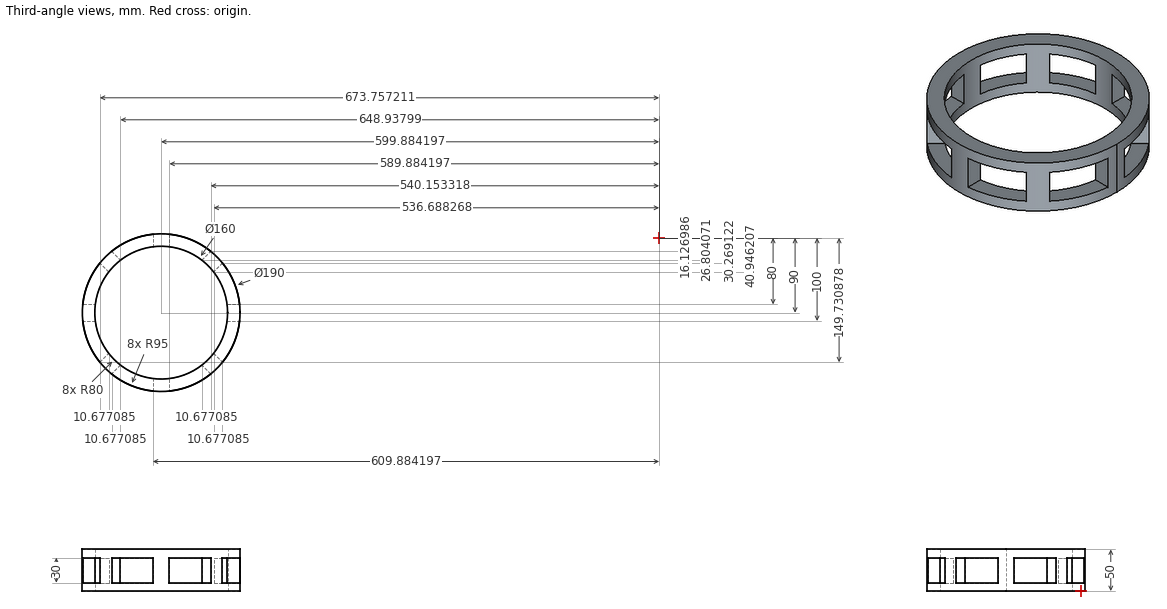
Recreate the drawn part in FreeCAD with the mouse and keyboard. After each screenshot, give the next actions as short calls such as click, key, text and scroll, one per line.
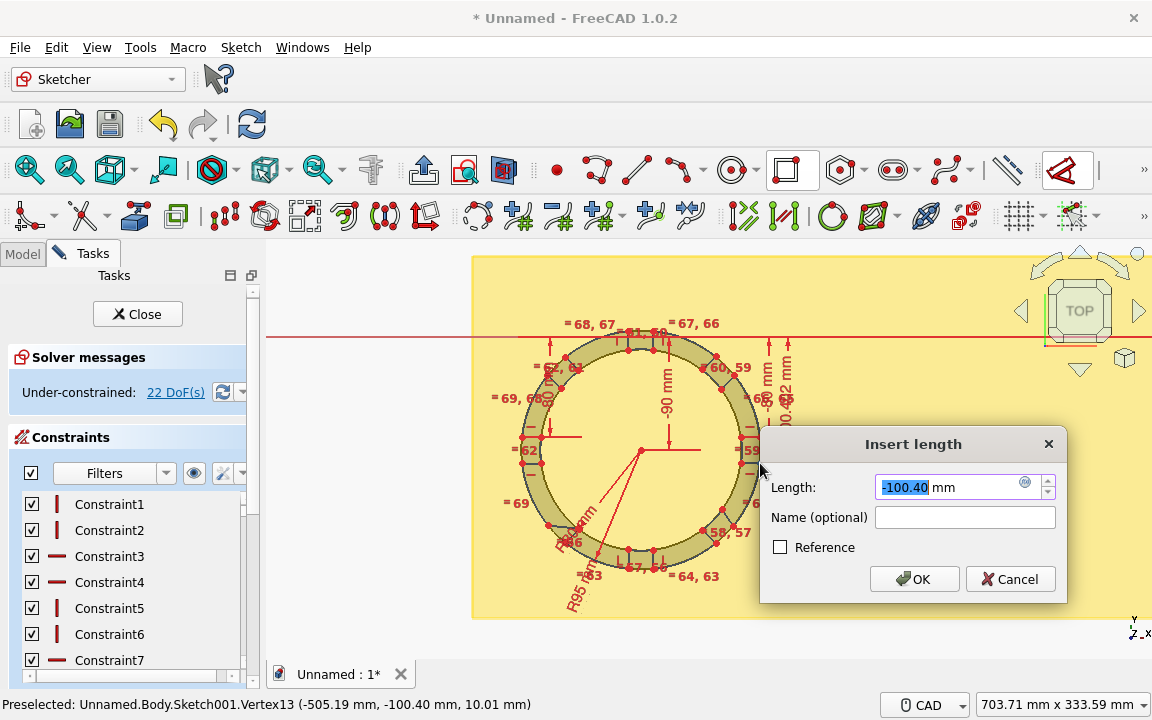
text(-100)
key(Return)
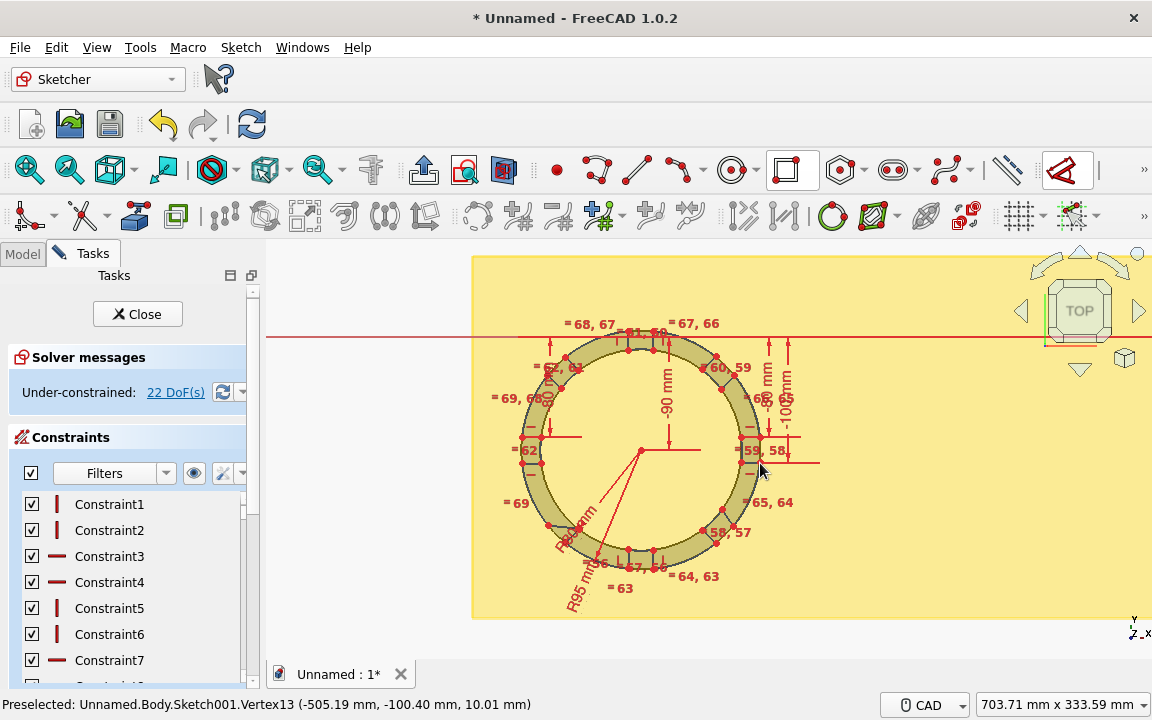
click(541, 464)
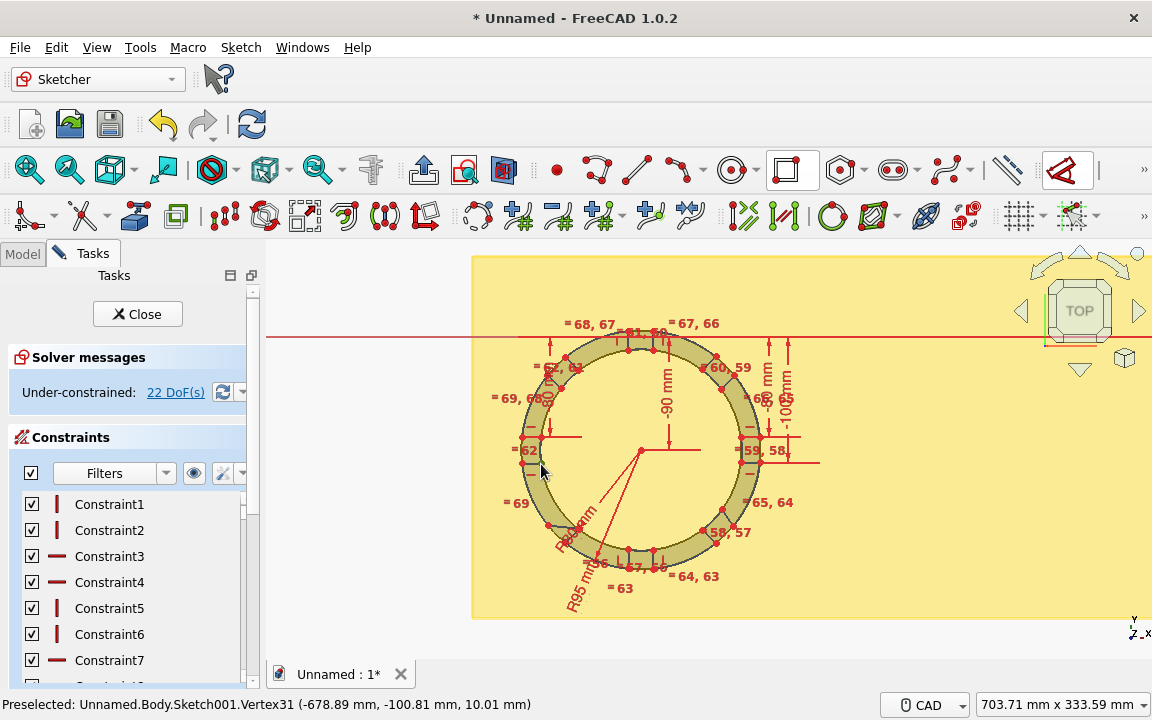
key(i)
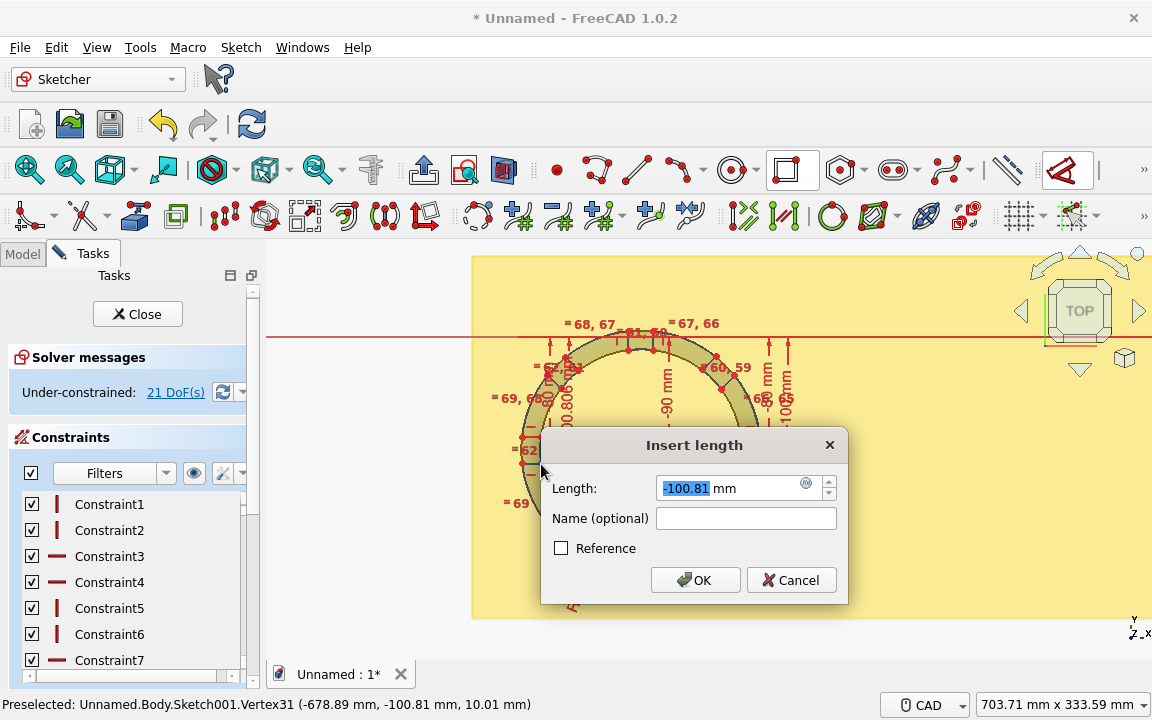
text(-100)
key(Return)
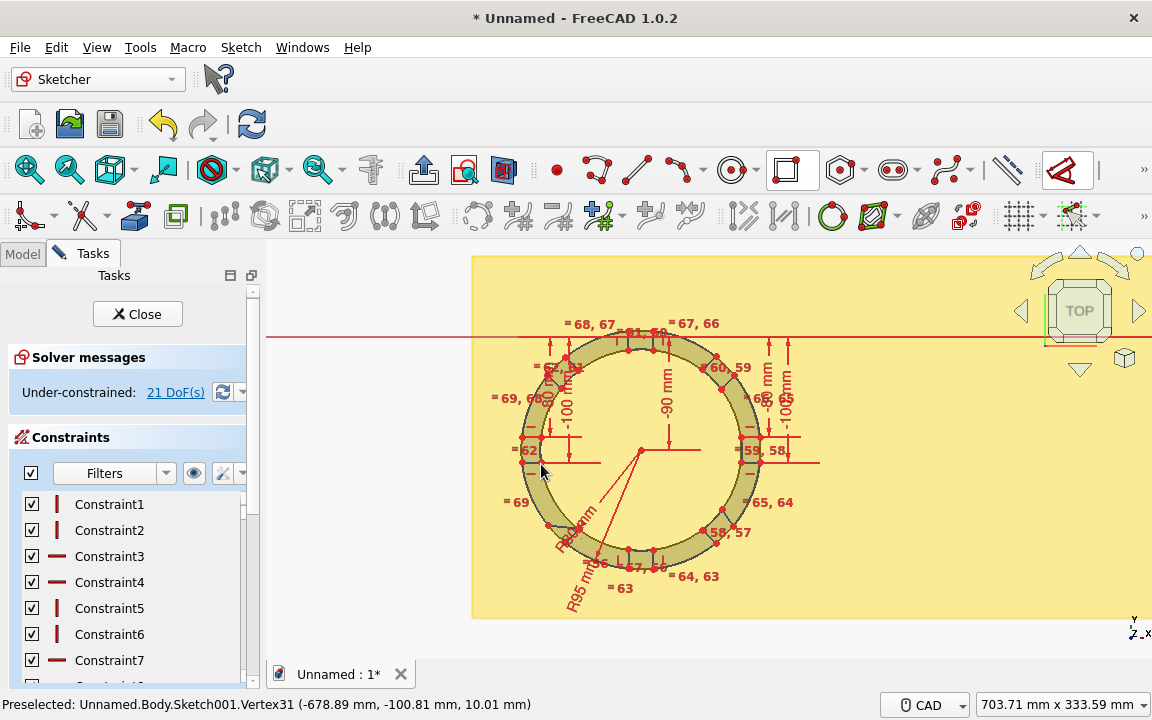
scroll(579, 530, up, 11)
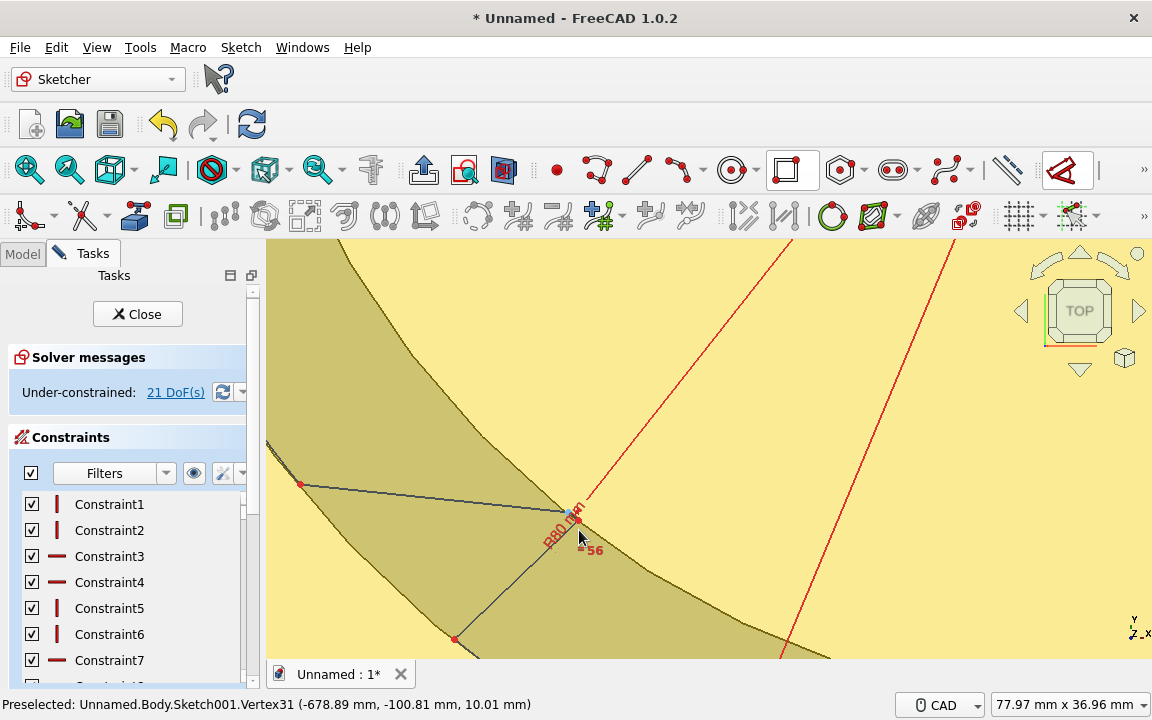
click(579, 520)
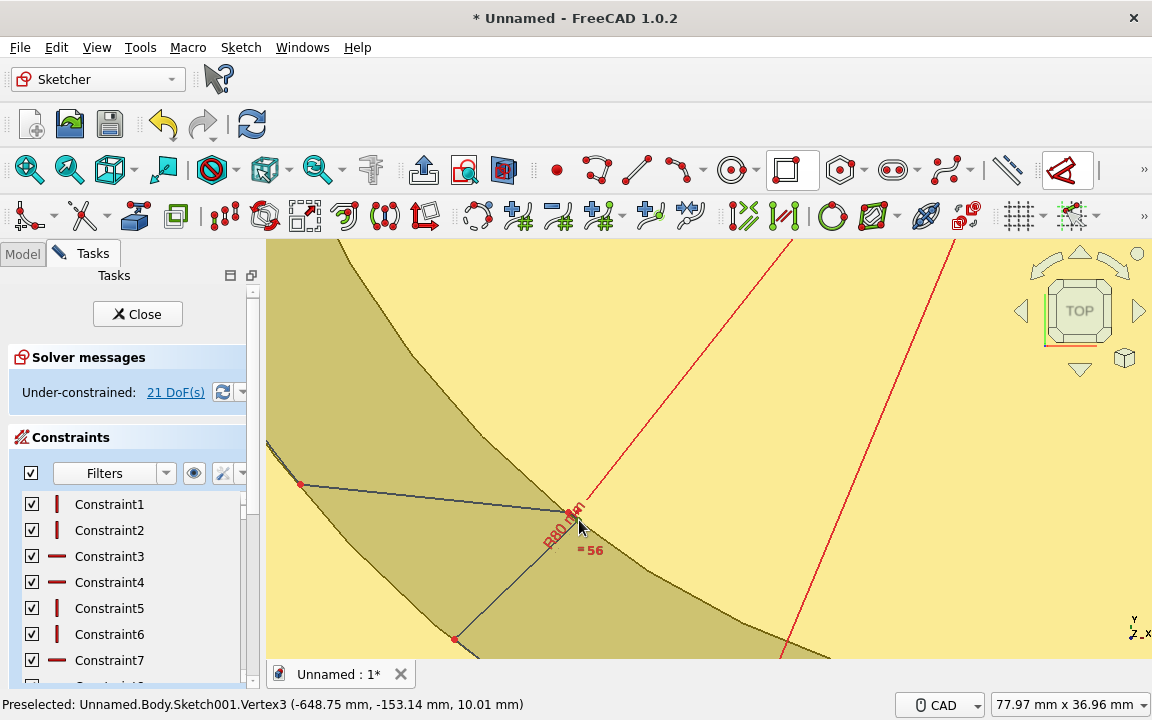
key(l)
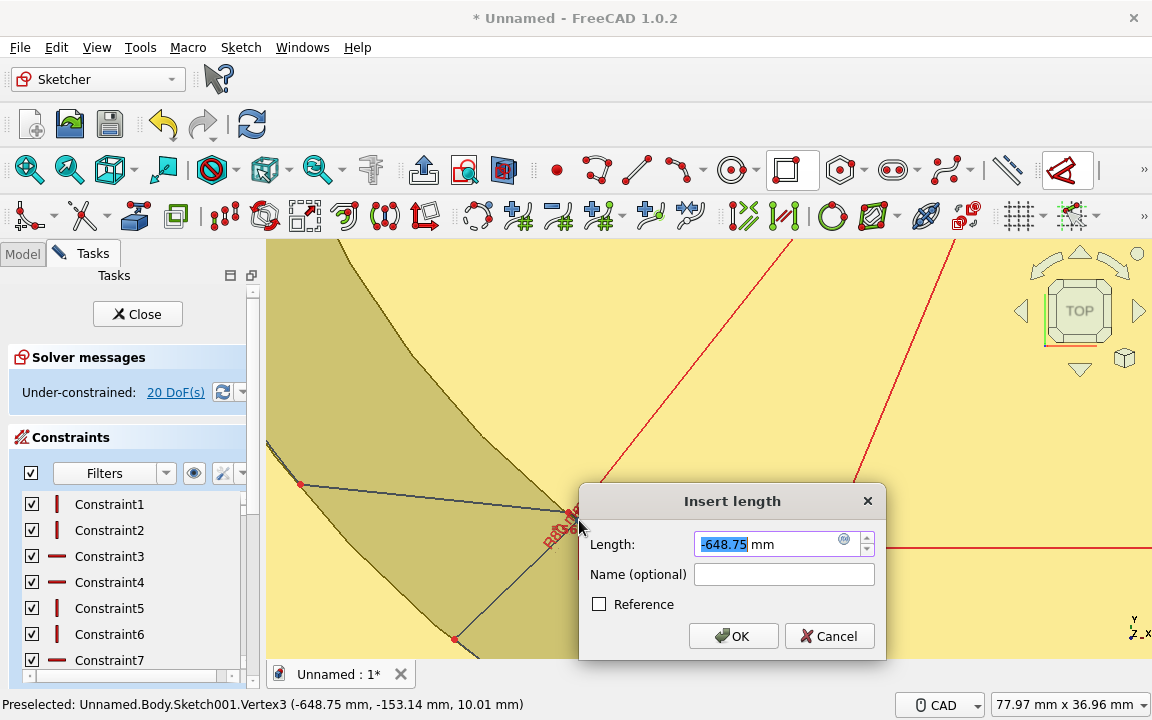
text(-648.93799)
key(Return)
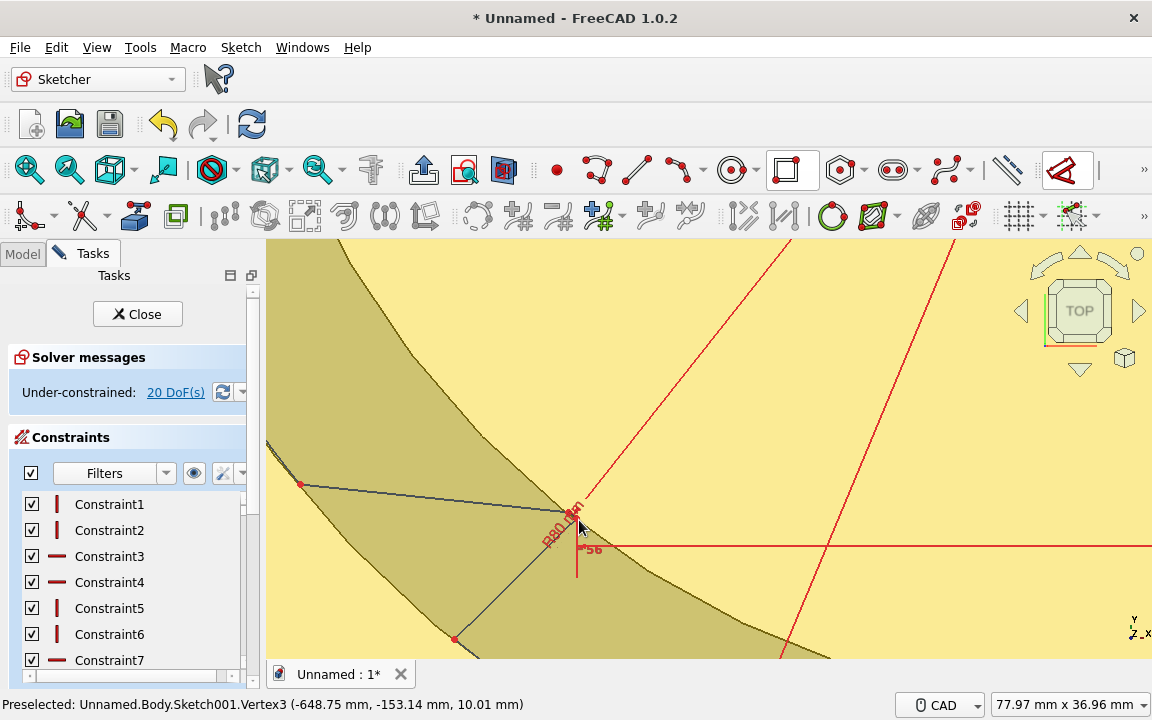
scroll(579, 530, down, 11)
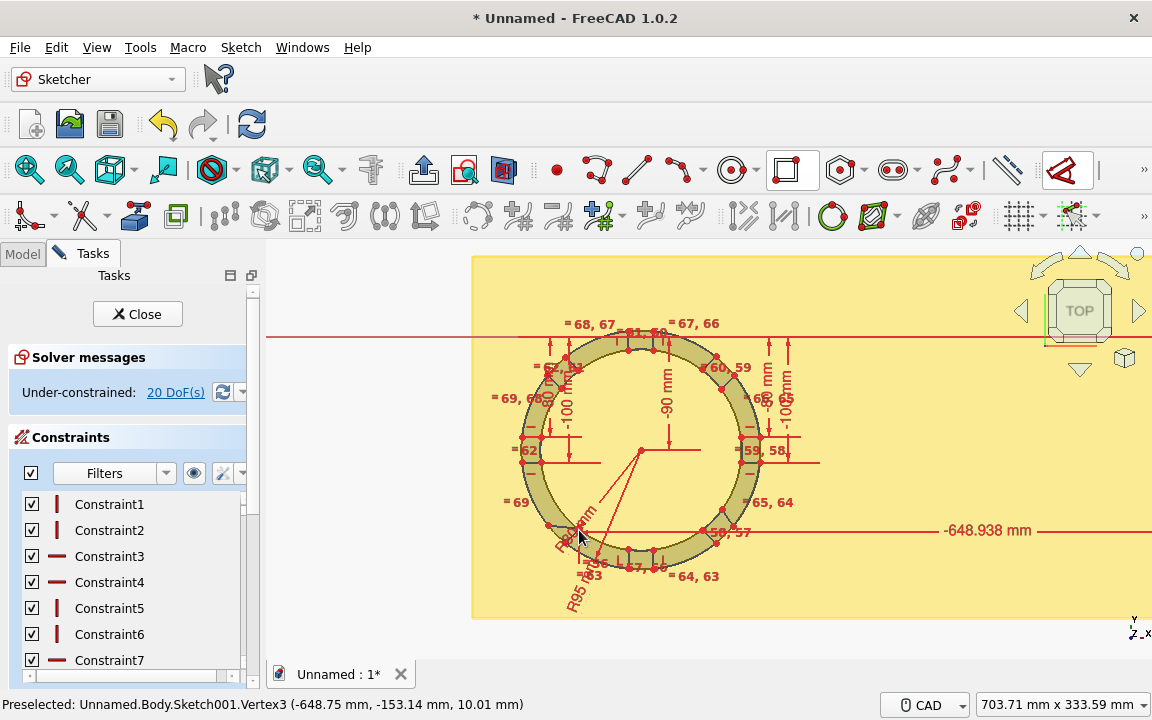
click(735, 376)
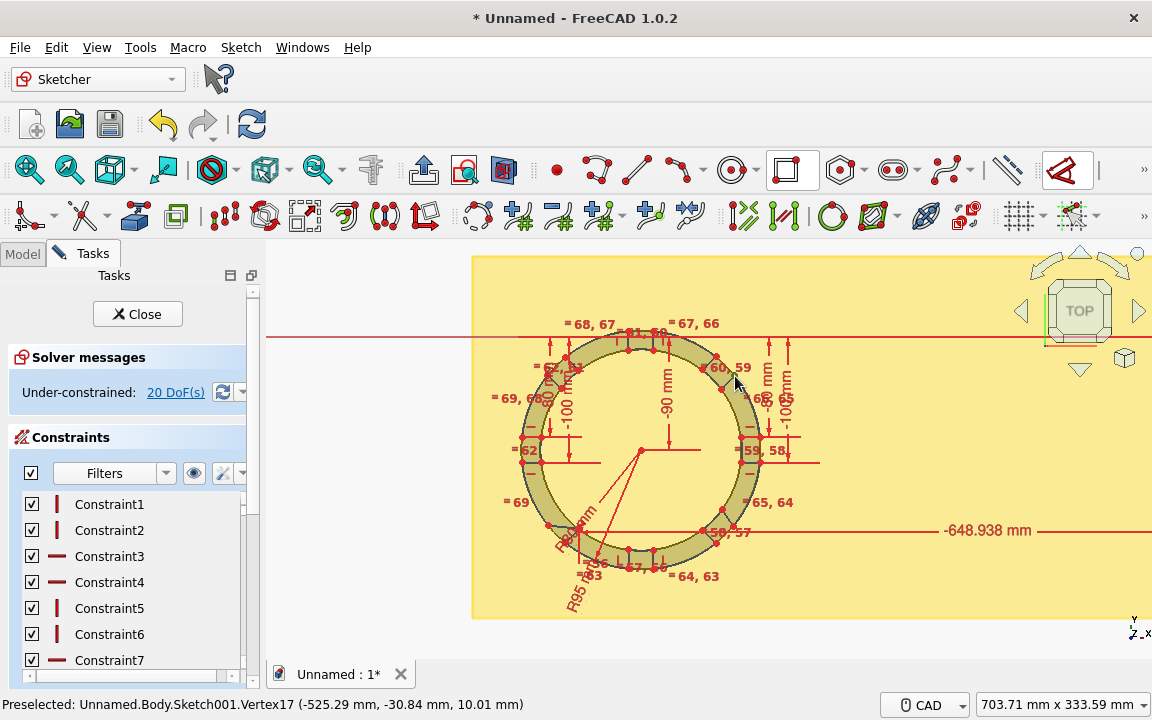
key(i)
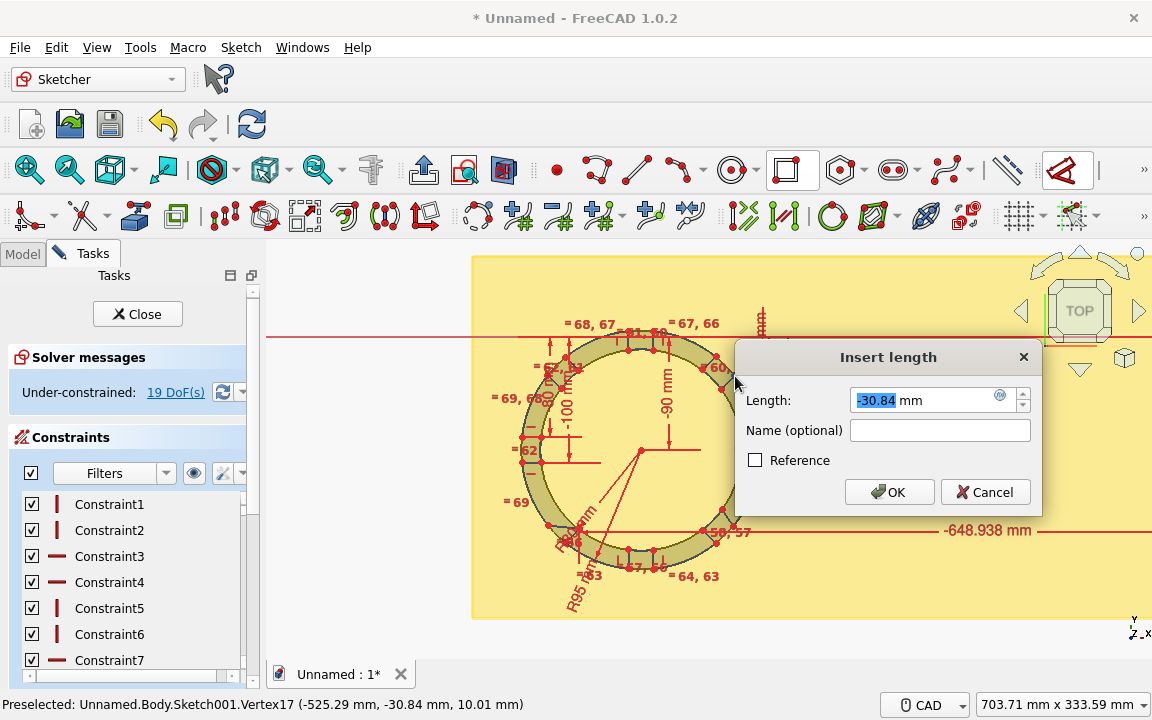
text(-30.269122)
key(Return)